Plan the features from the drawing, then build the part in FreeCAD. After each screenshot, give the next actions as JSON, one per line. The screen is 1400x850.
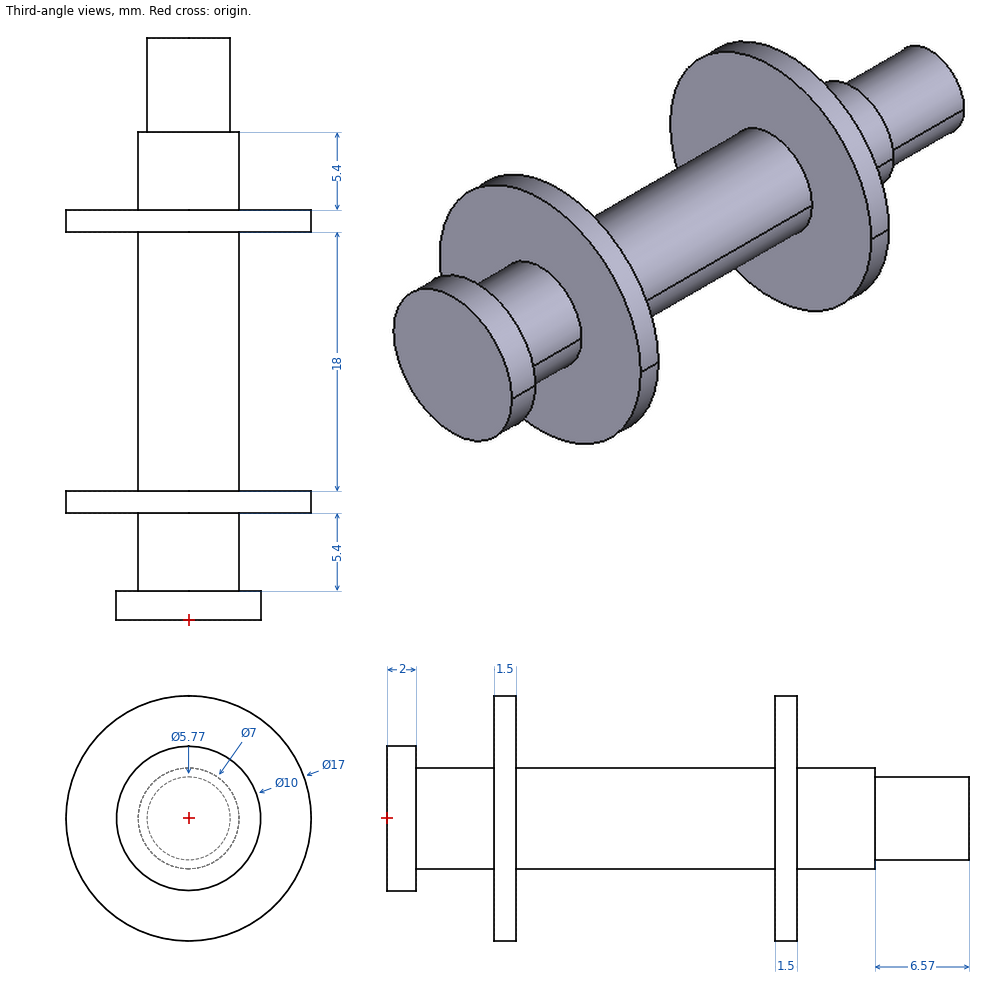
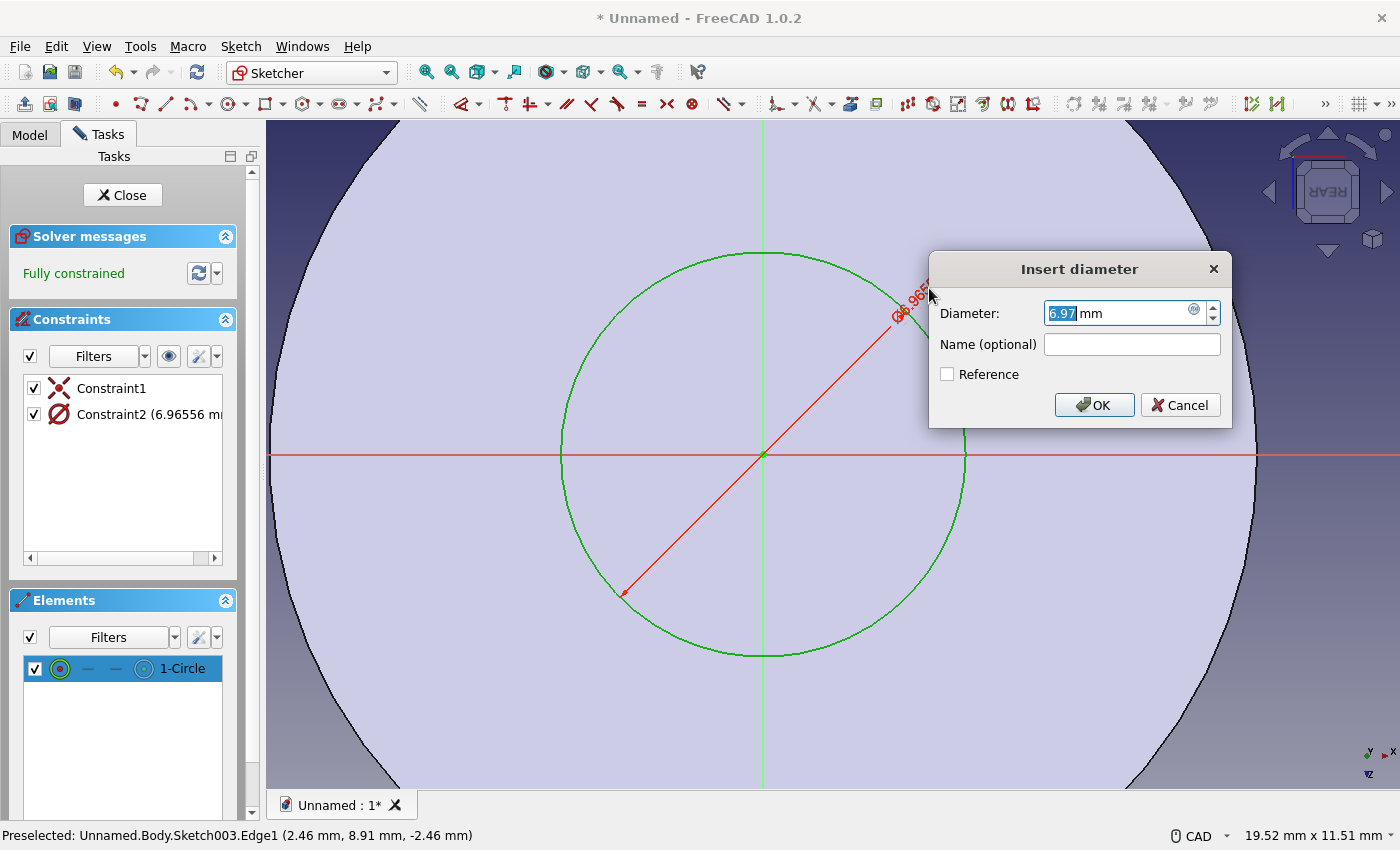
{"action": "type", "text": "7"}
{"action": "key", "text": "Return"}
{"action": "key", "text": "Escape"}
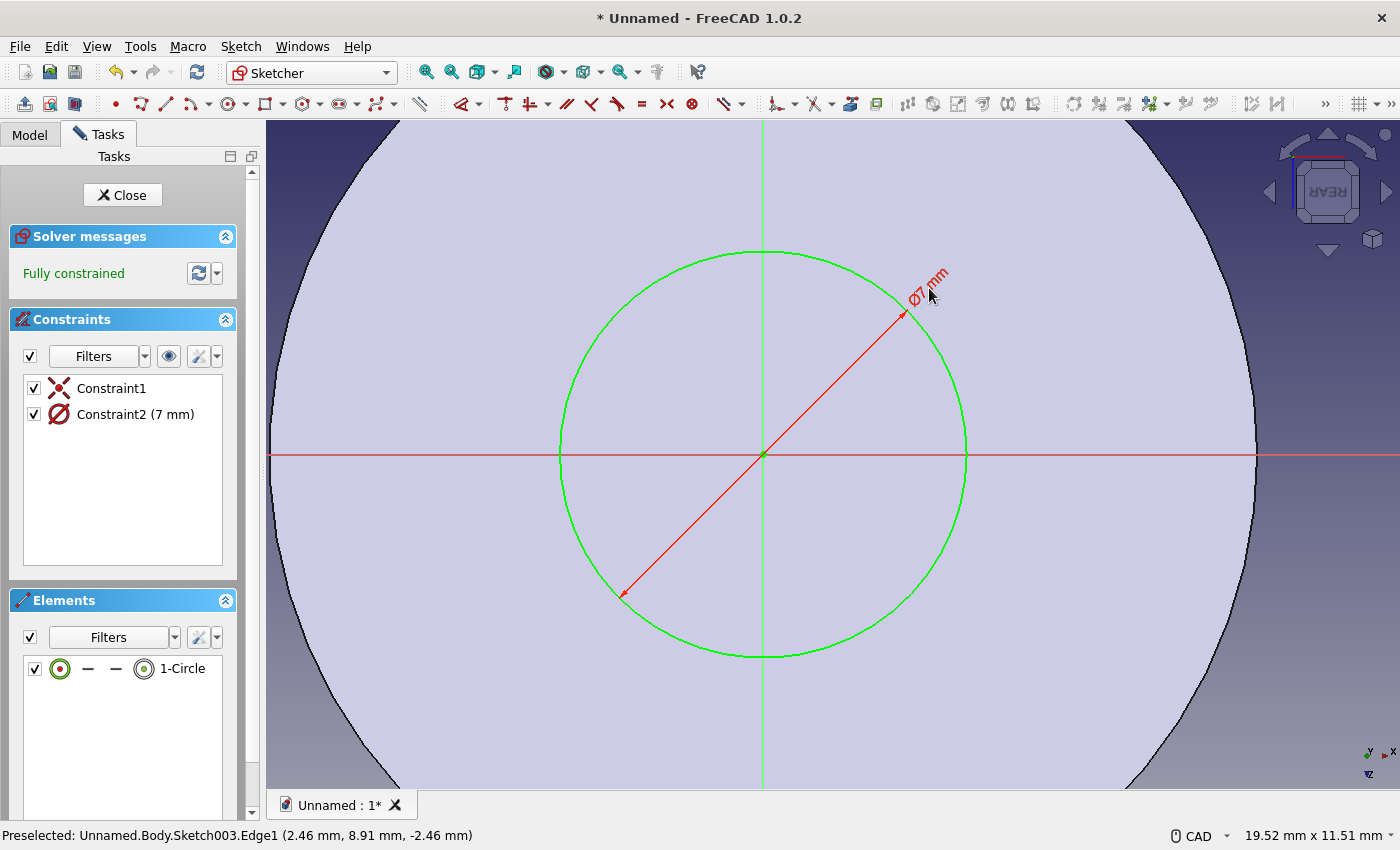
{"action": "left_click", "coordinate": [123, 195]}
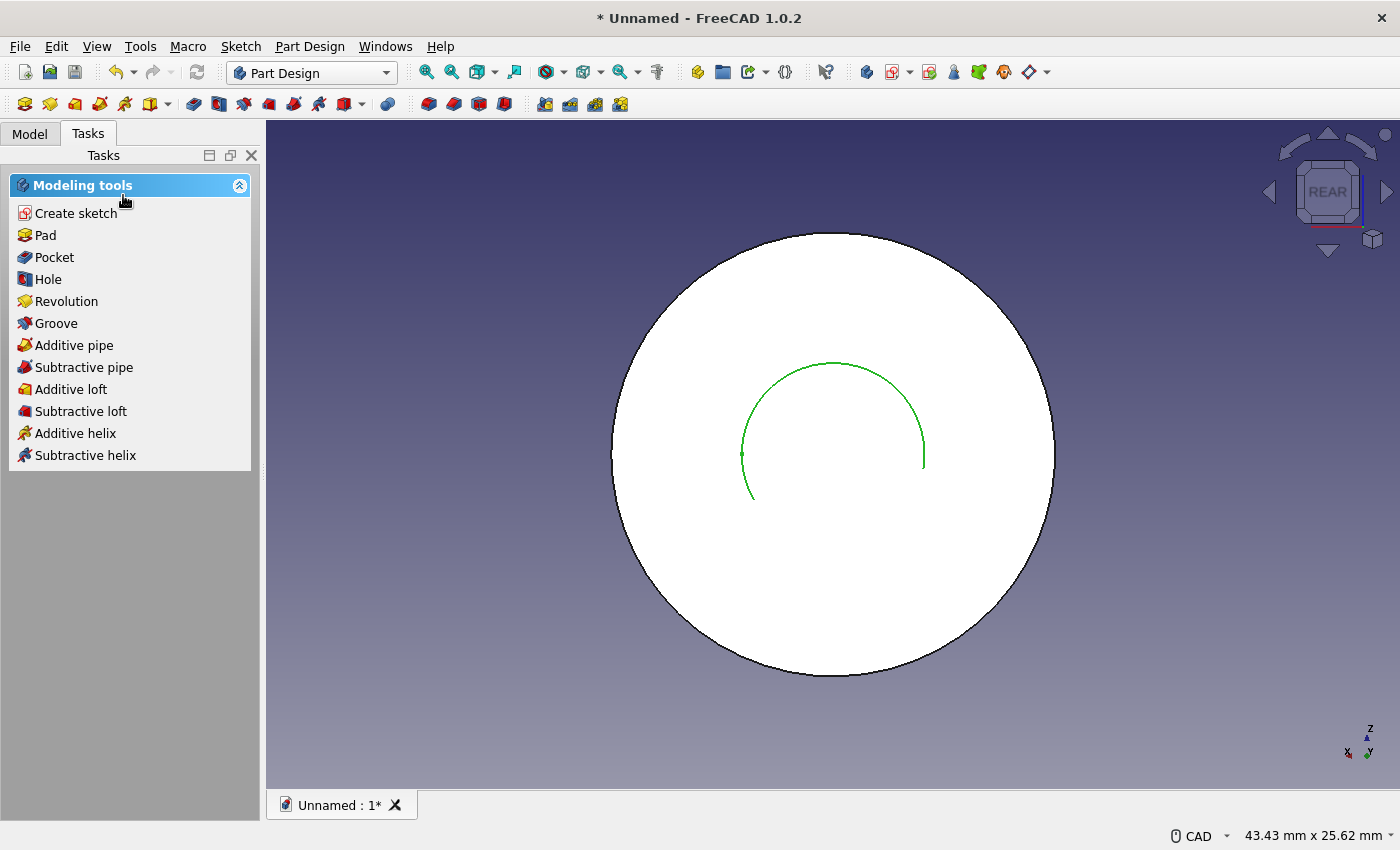
{"action": "left_click", "coordinate": [25, 104]}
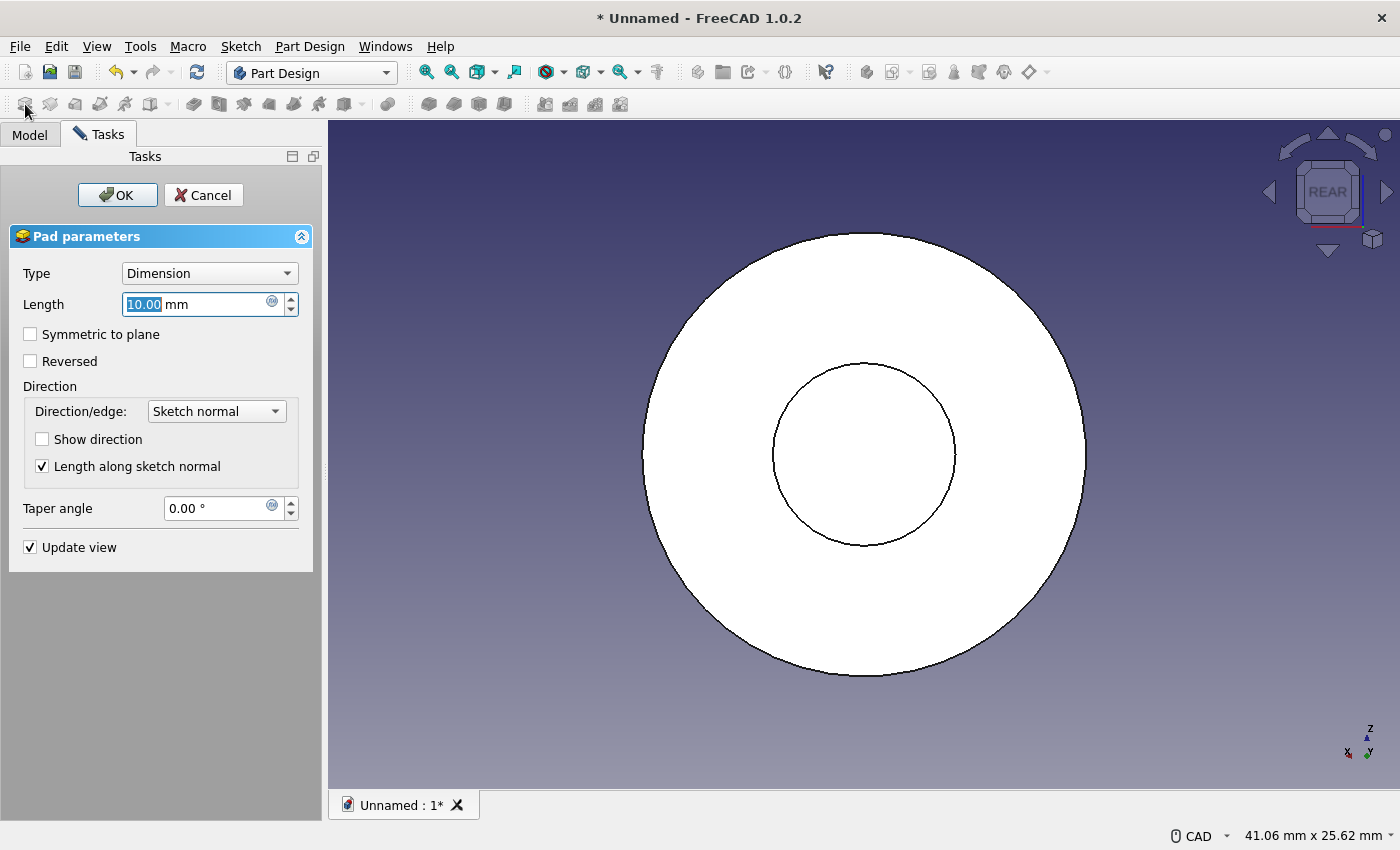
{"action": "type", "text": "18"}
{"action": "key", "text": "Tab"}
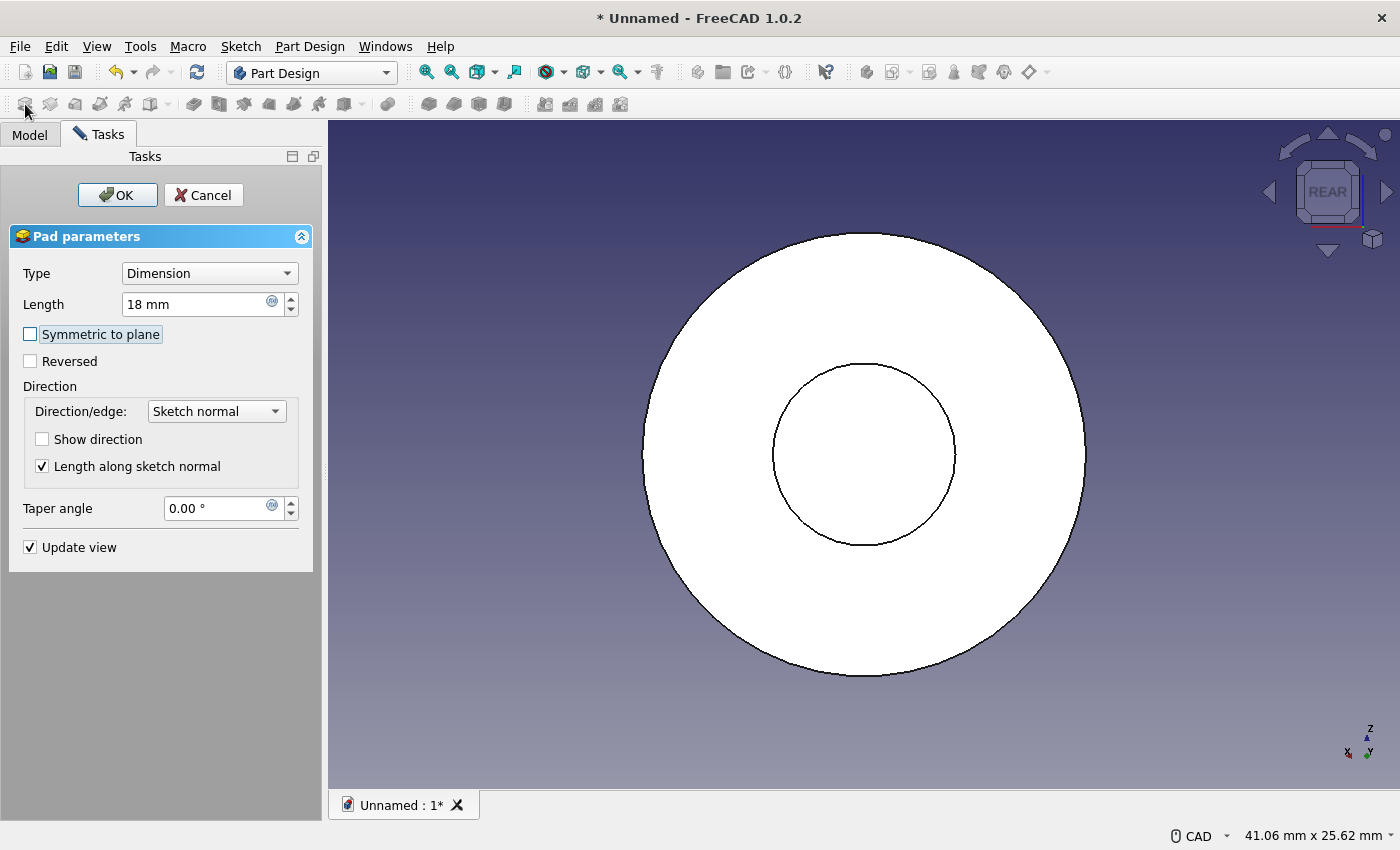
{"action": "left_click", "coordinate": [118, 195]}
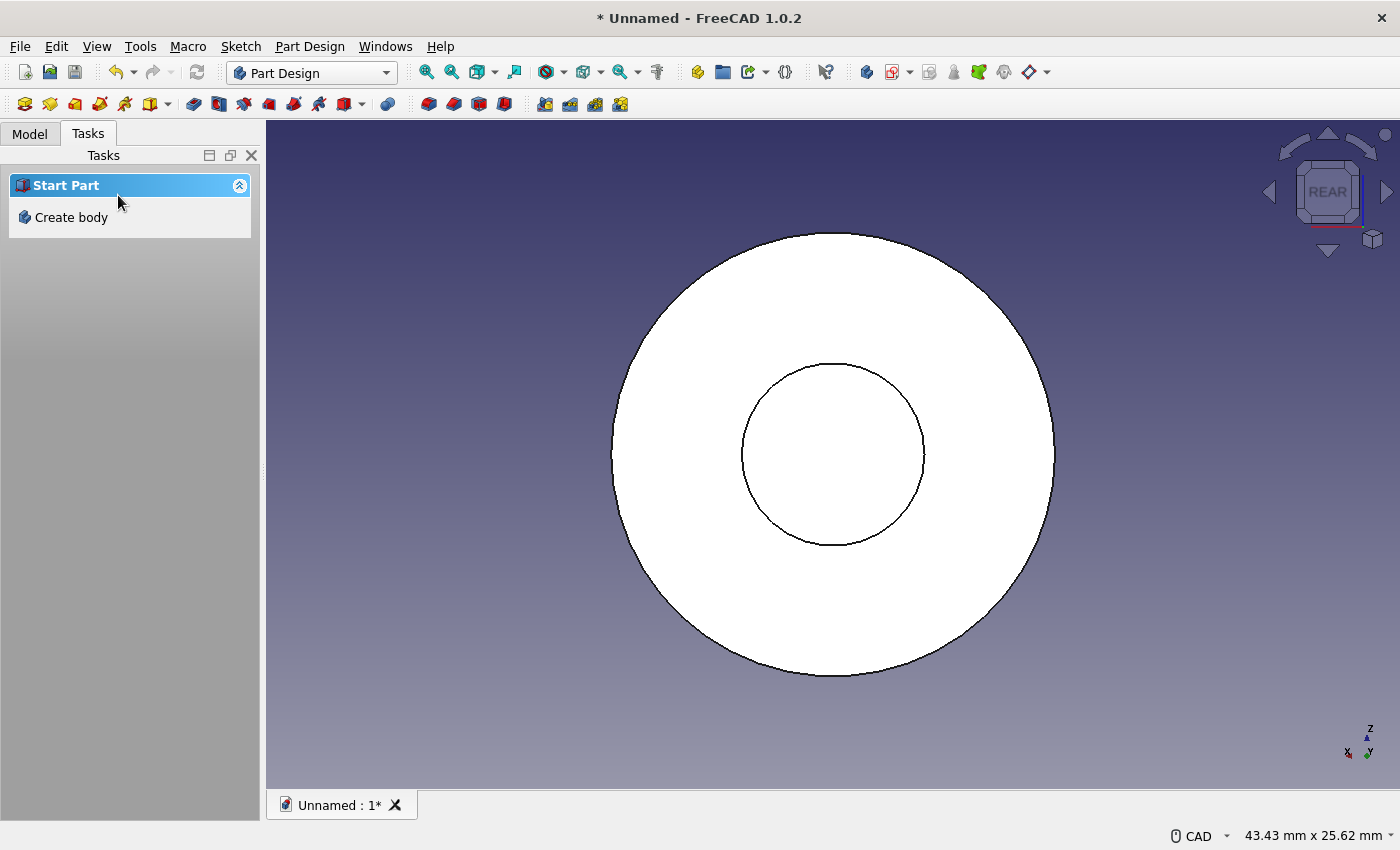
{"action": "left_click", "coordinate": [833, 453]}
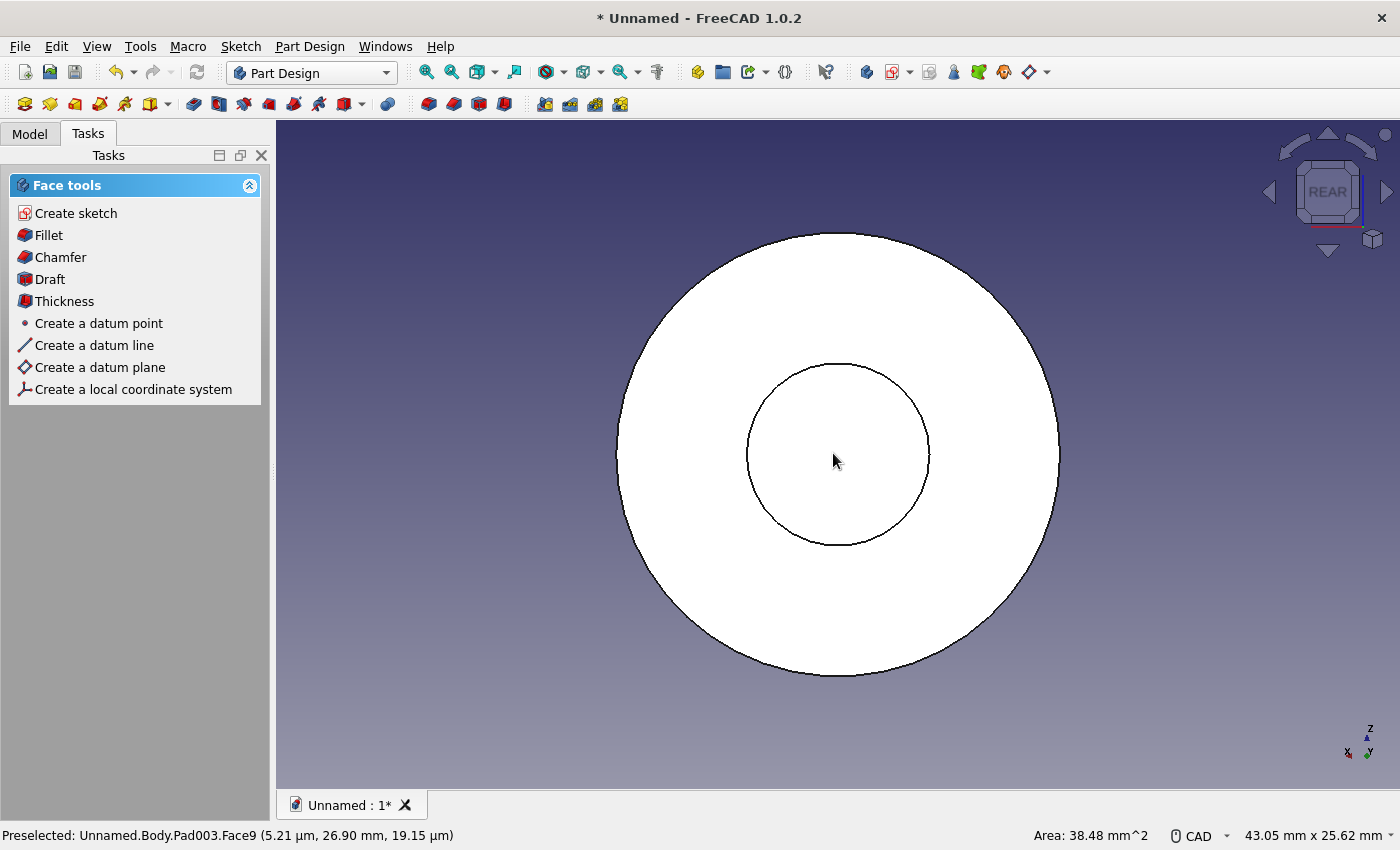
{"action": "left_click", "coordinate": [892, 72]}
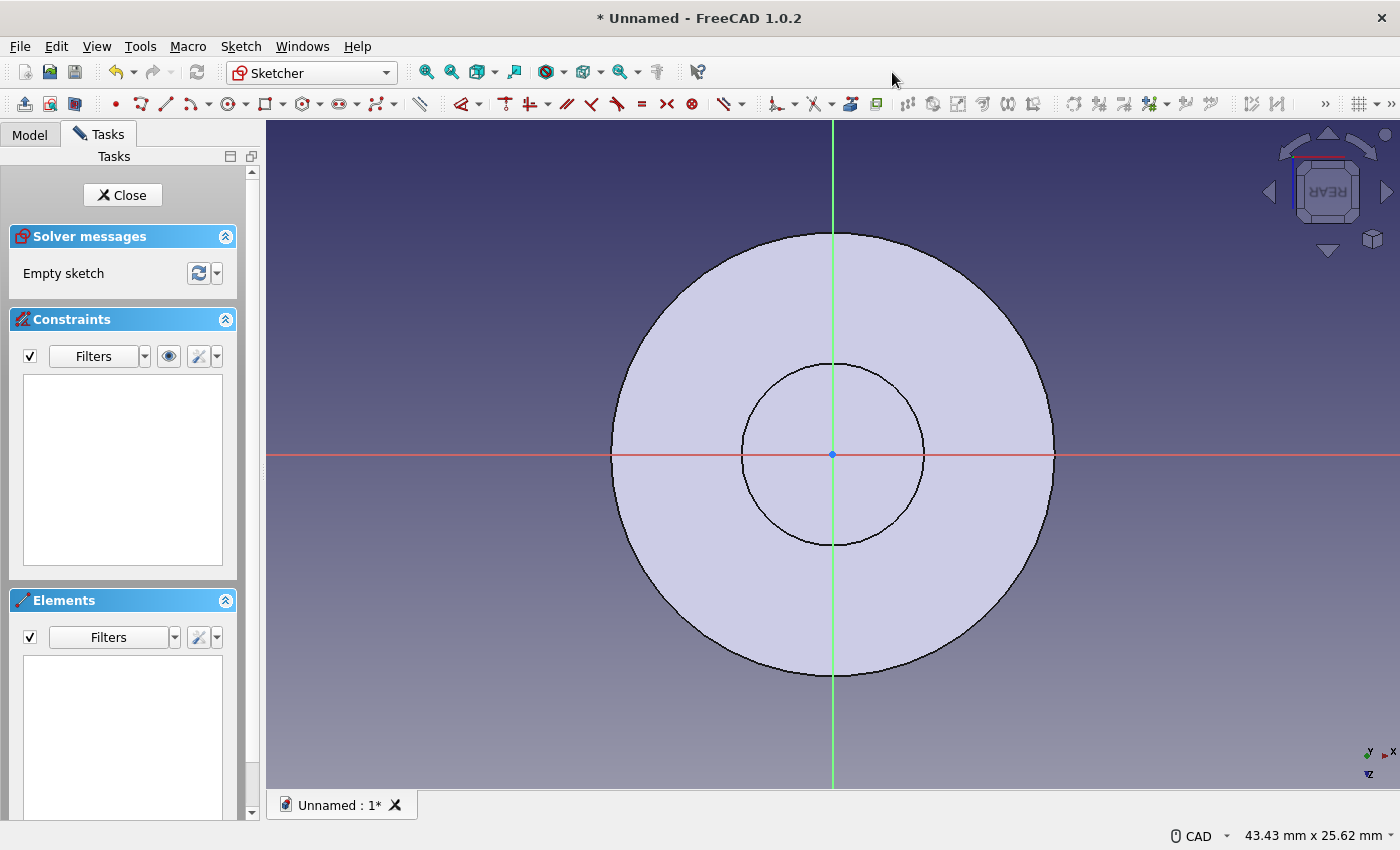
{"action": "left_click", "coordinate": [228, 104]}